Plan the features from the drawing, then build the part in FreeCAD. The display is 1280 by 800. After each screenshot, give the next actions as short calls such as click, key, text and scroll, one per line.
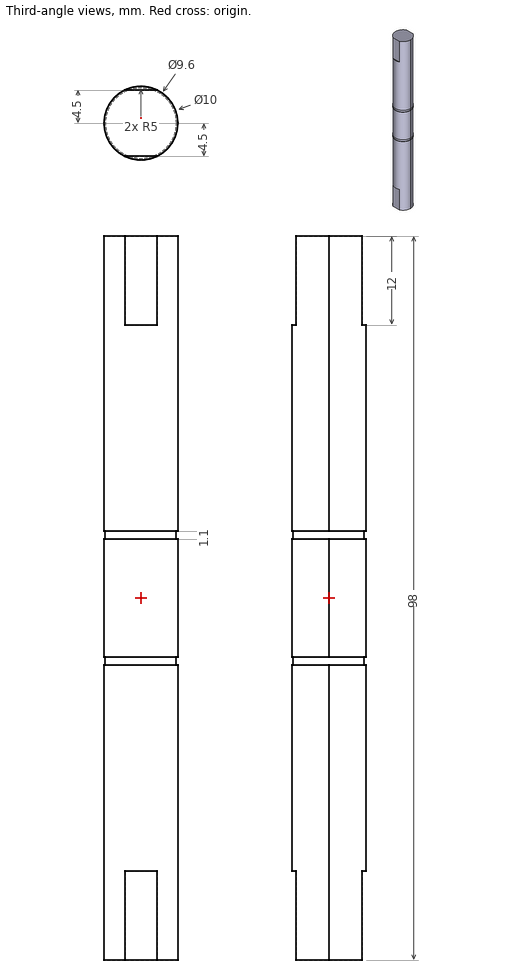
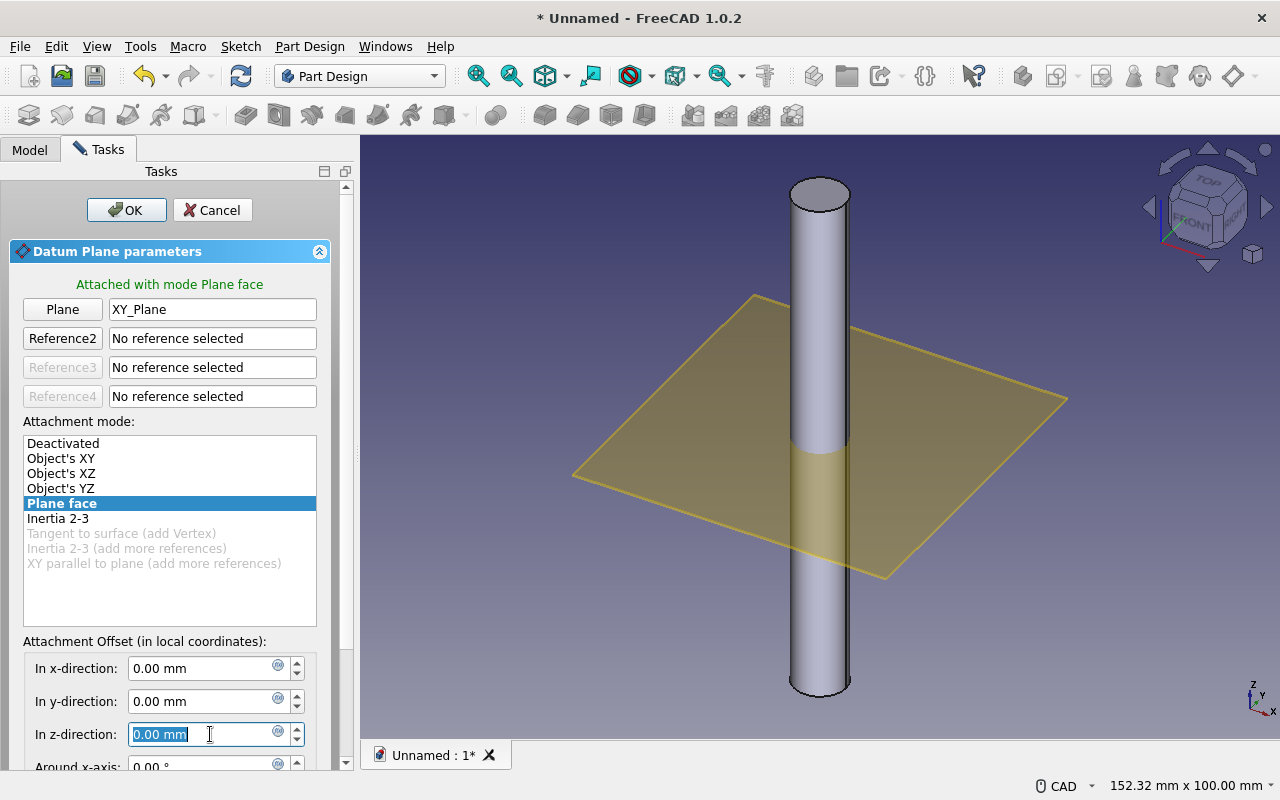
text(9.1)
key(Tab)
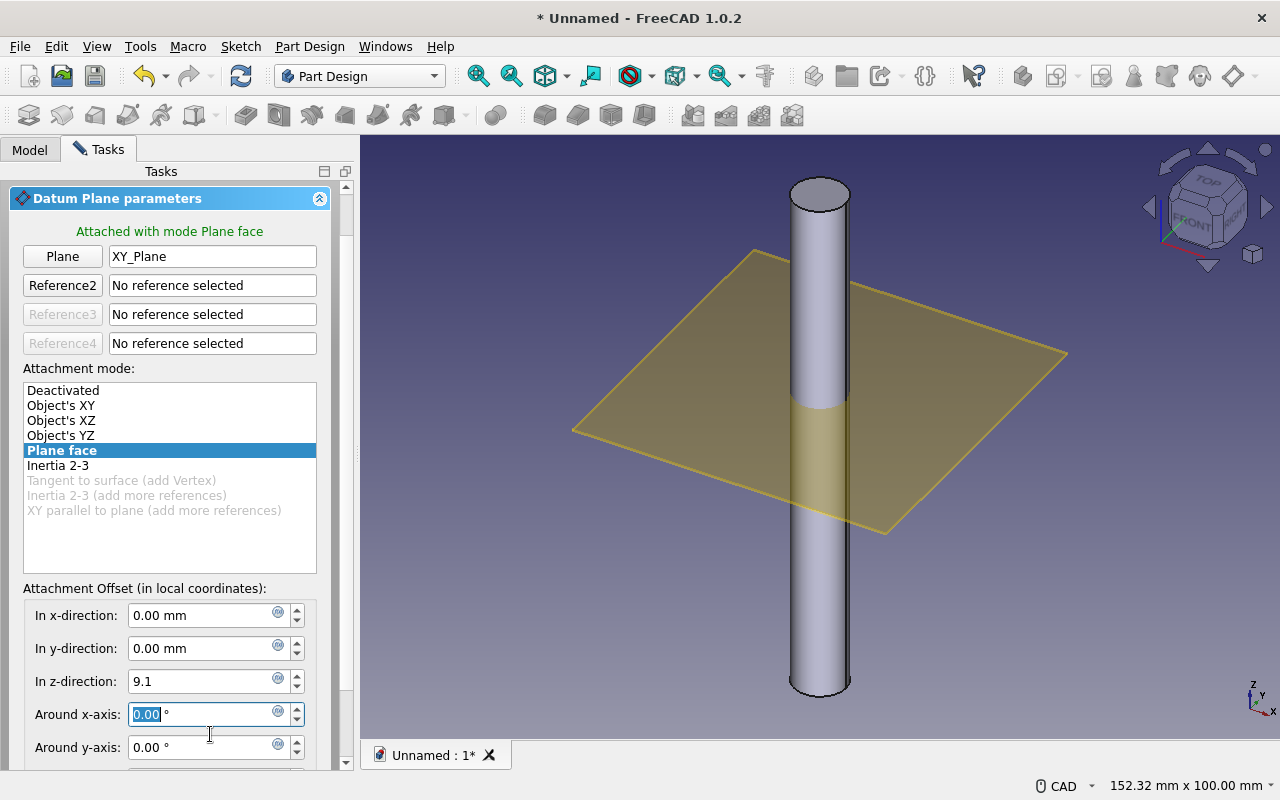
scroll(346, 476, up, 2)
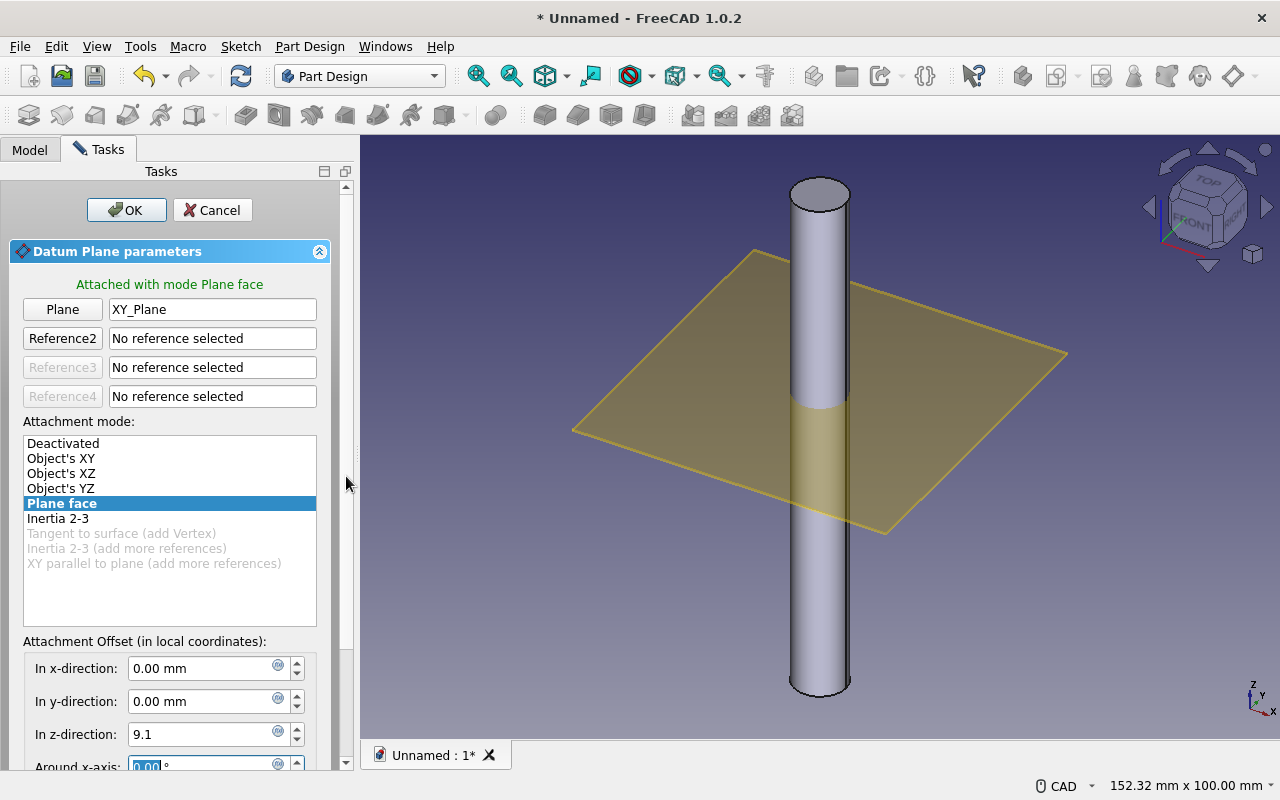
click(127, 210)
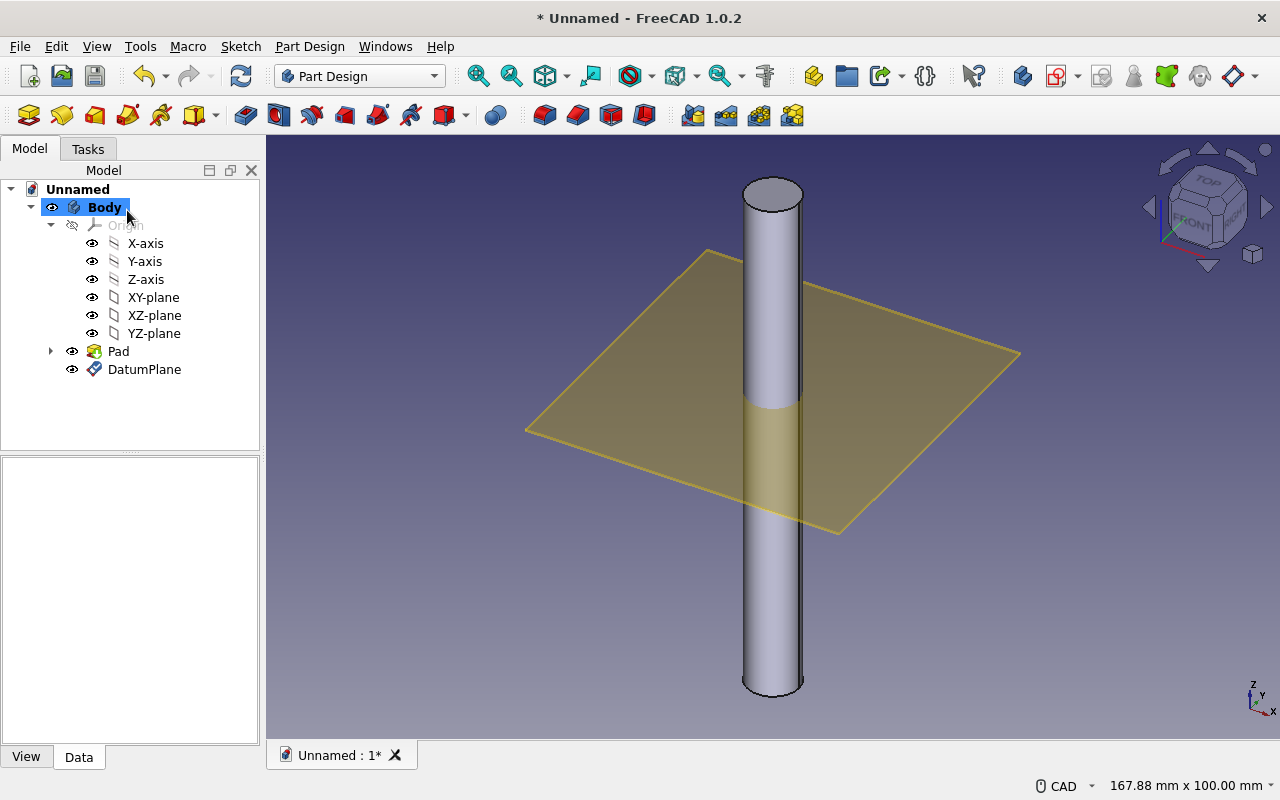
click(117, 369)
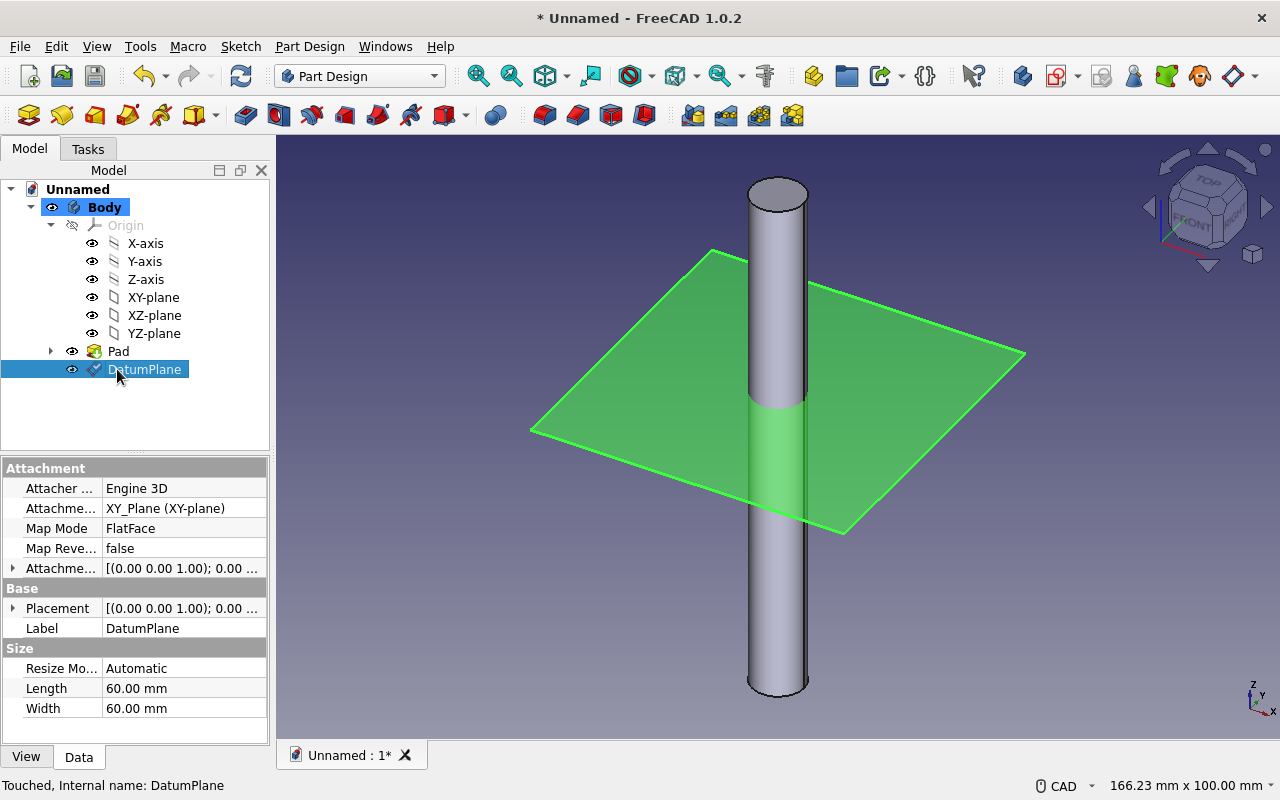
click(1056, 76)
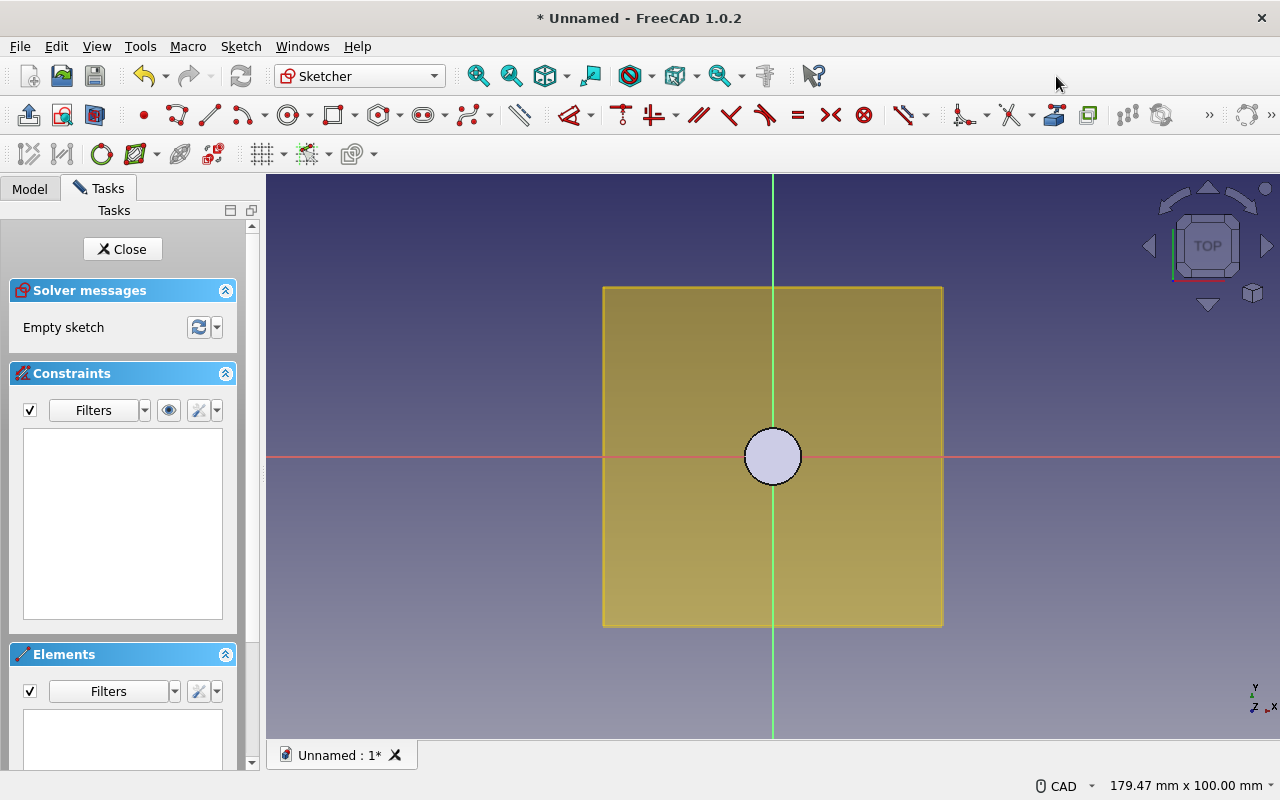
click(95, 116)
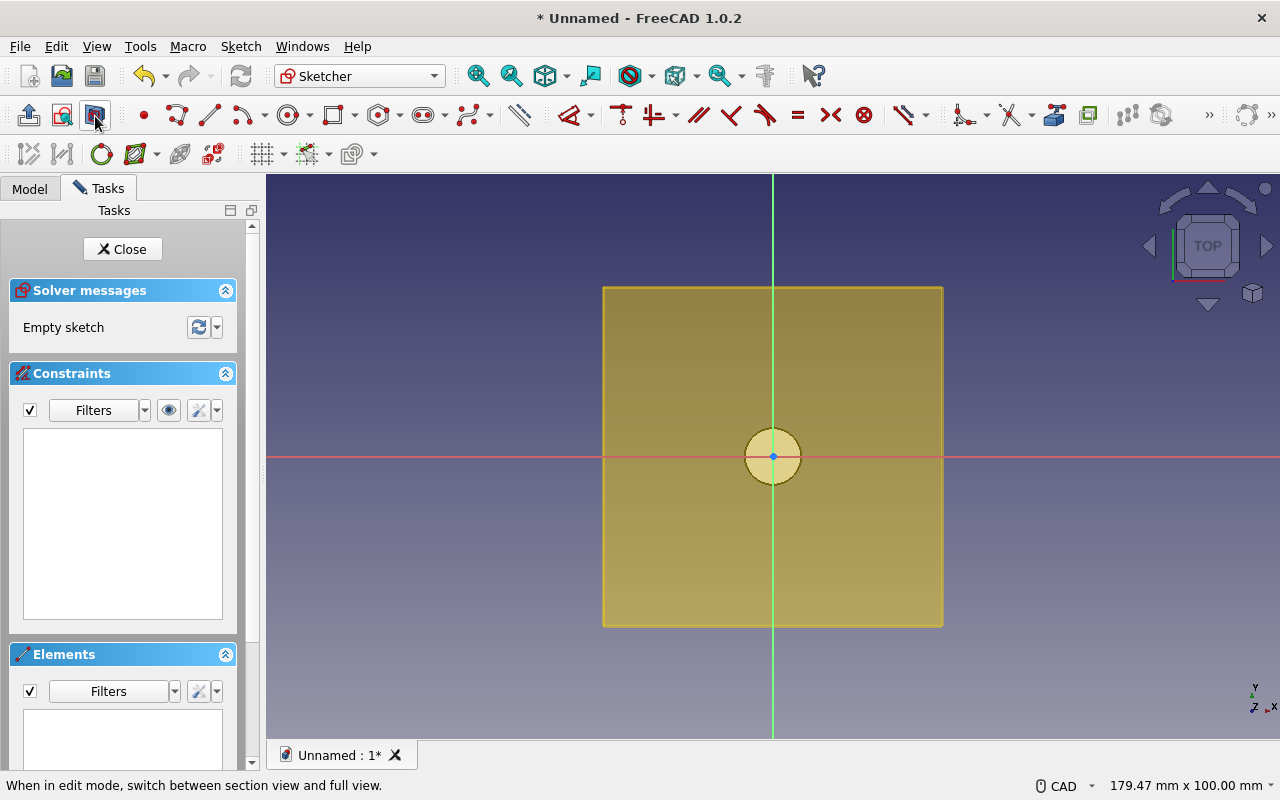
scroll(787, 456, up, 9)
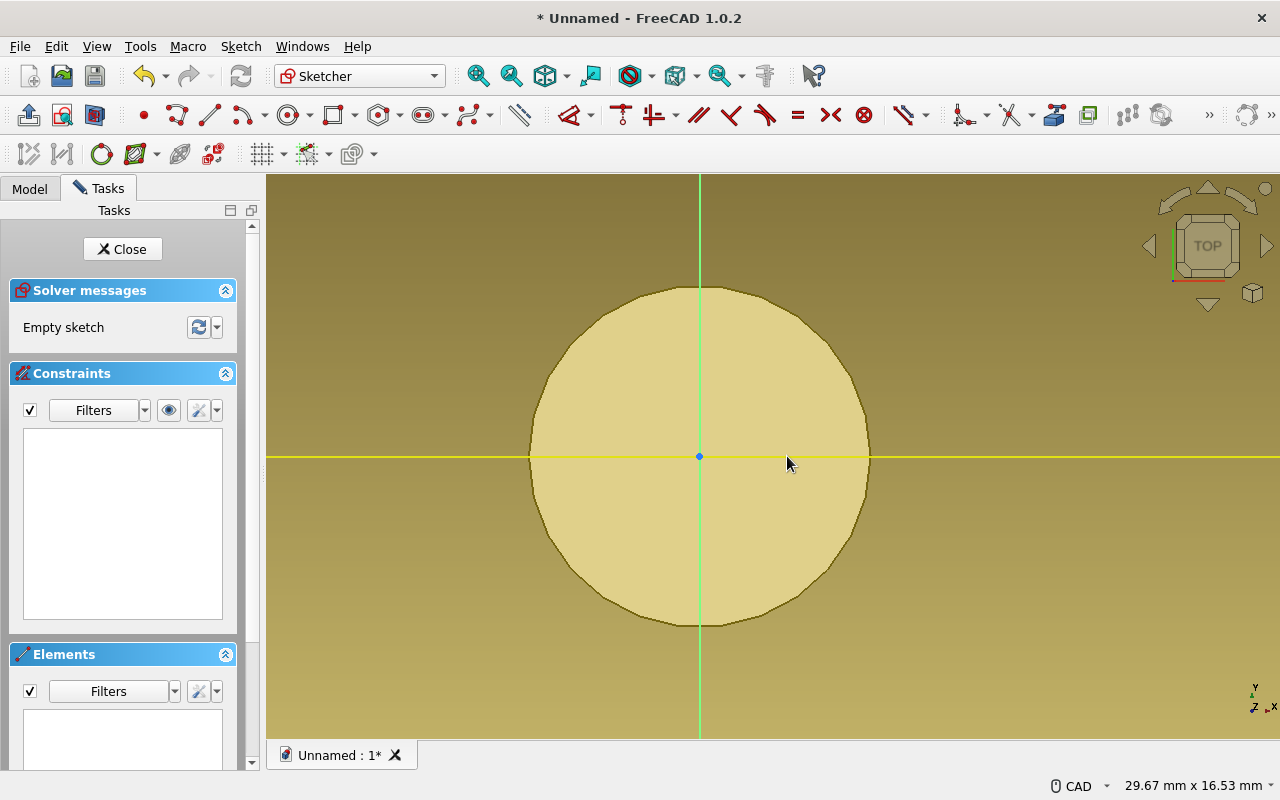
click(288, 116)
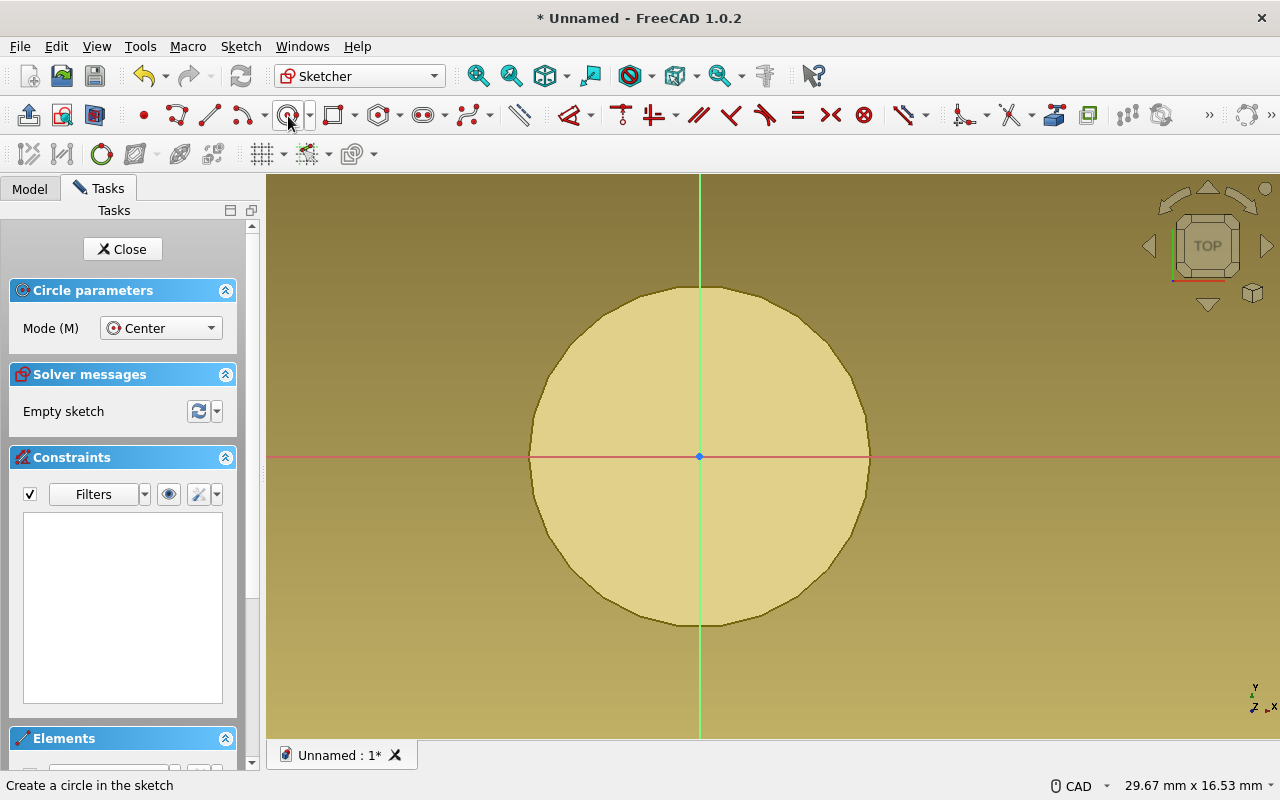
click(700, 456)
click(821, 336)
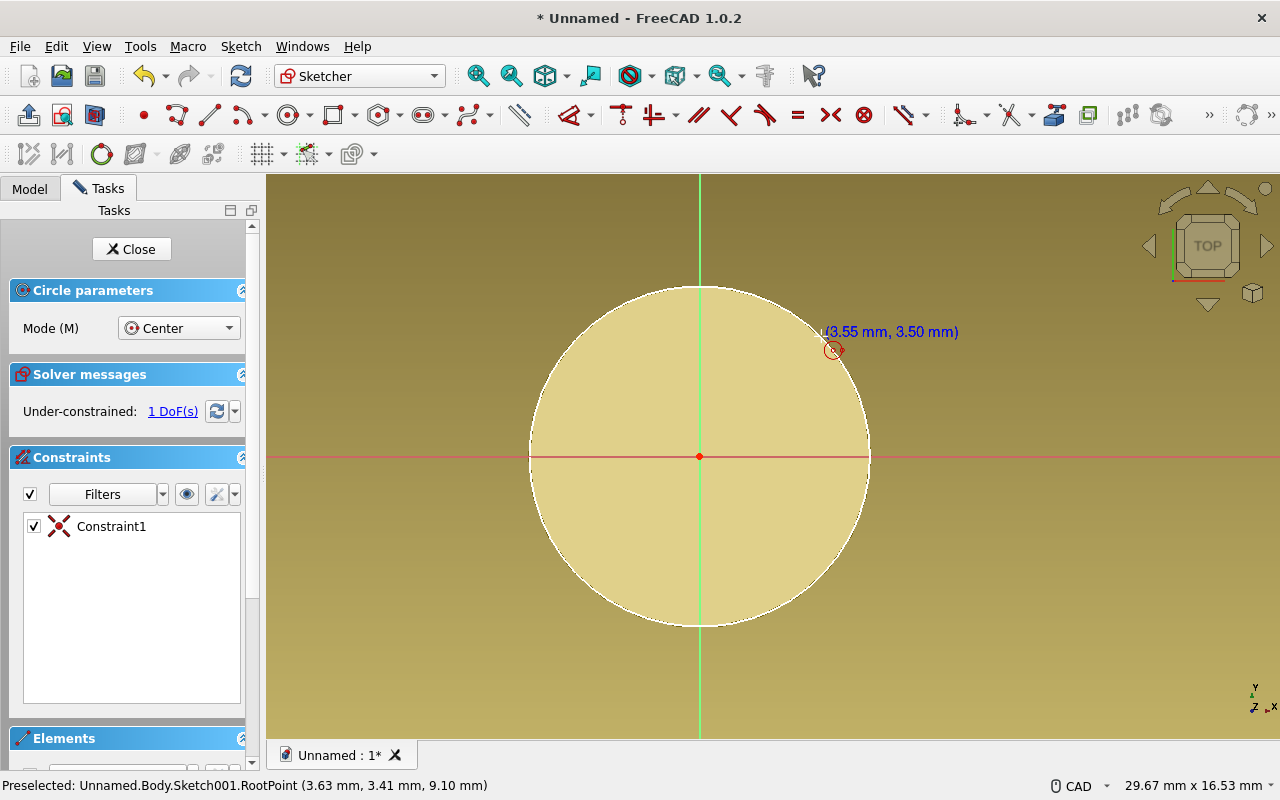
click(700, 456)